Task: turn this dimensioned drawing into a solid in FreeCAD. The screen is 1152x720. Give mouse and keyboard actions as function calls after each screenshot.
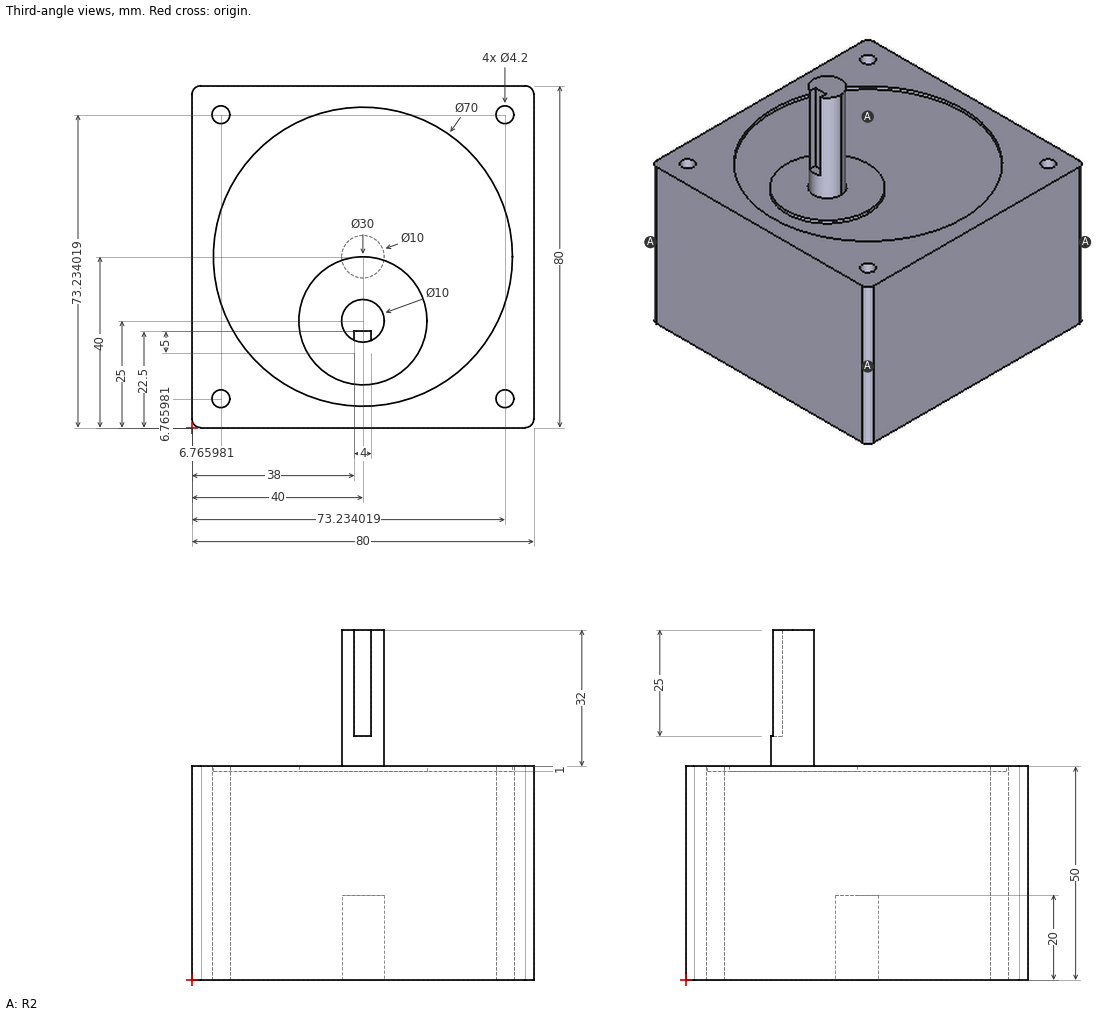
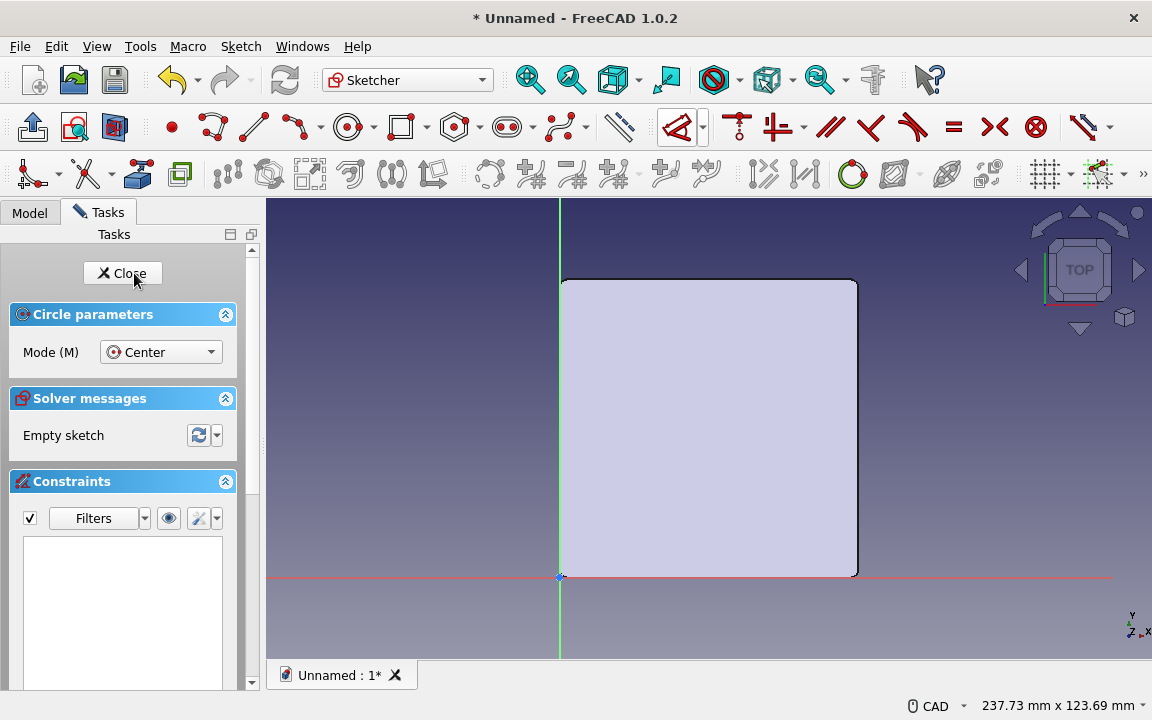
scroll(833, 305, up, 6)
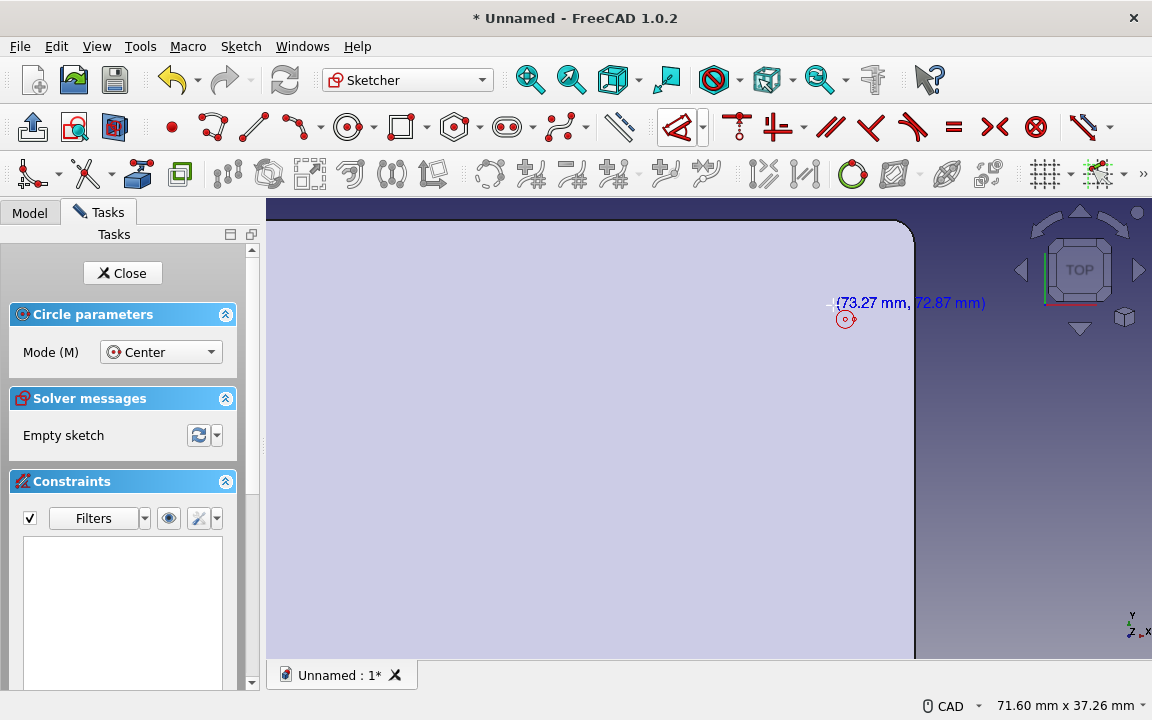
click(831, 303)
click(849, 285)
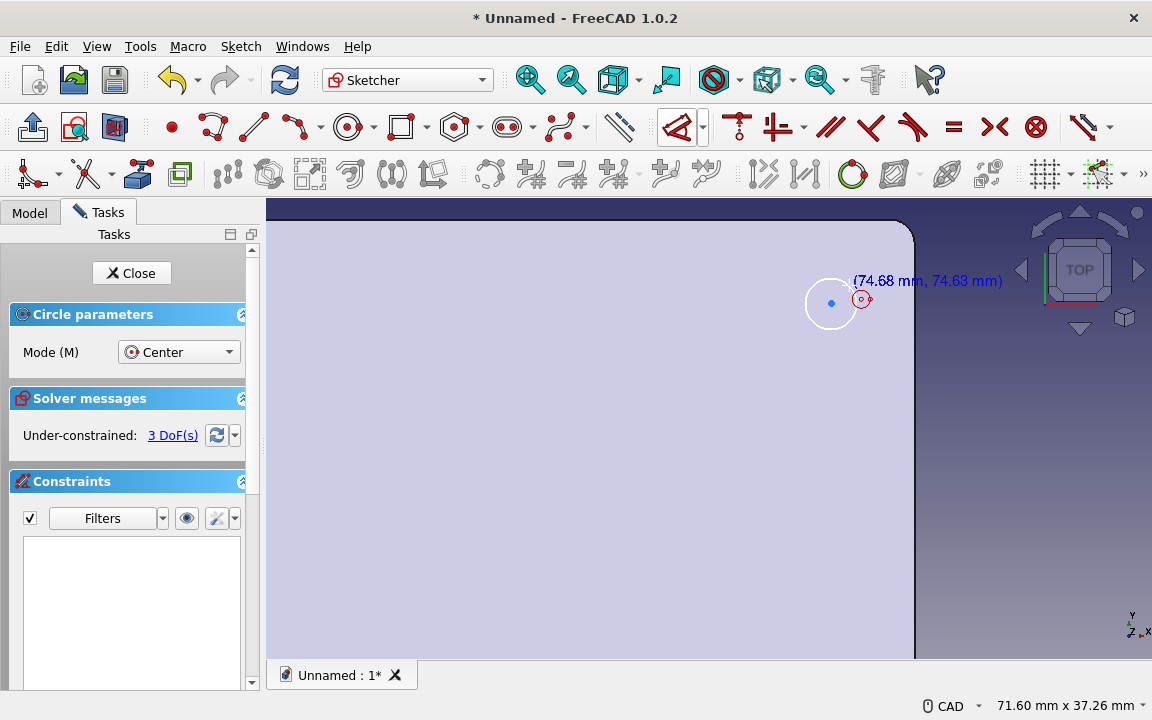
scroll(748, 293, down, 6)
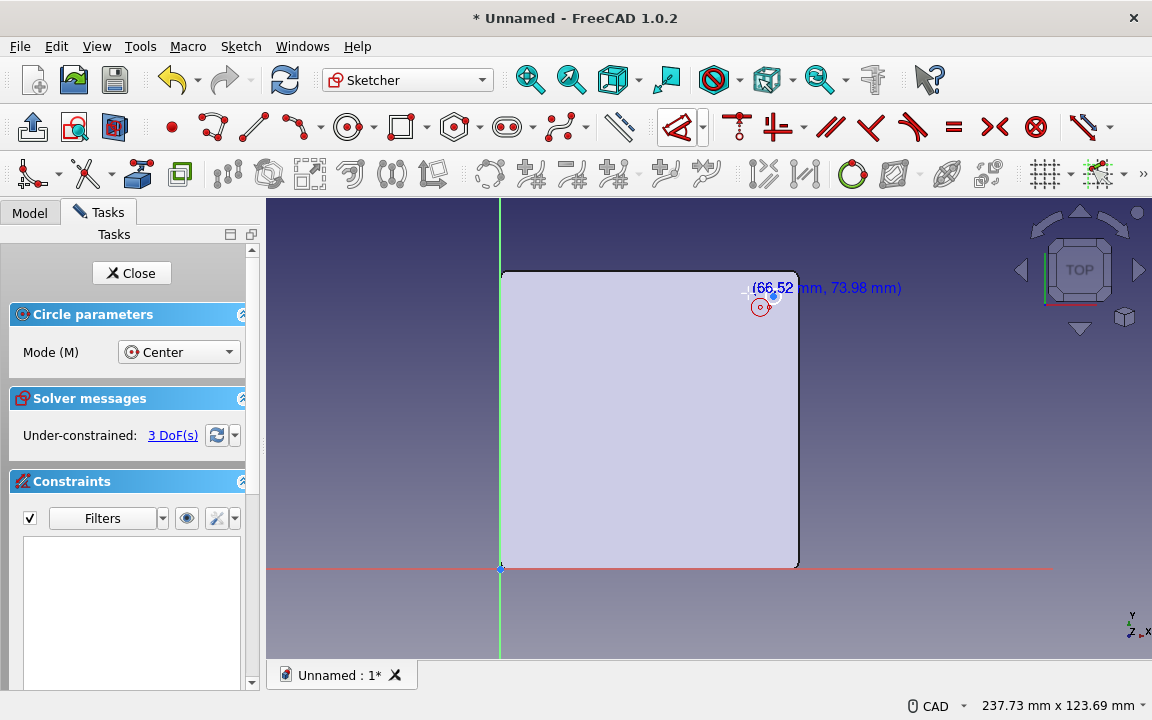
scroll(526, 296, up, 6)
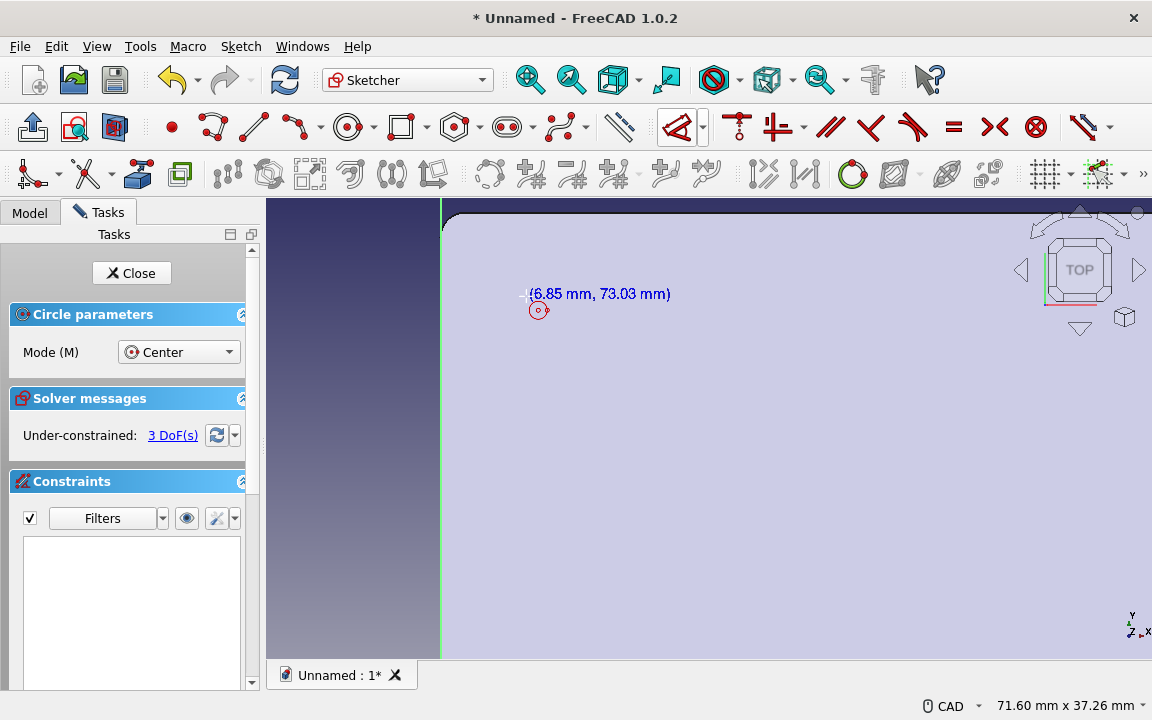
click(524, 296)
click(543, 278)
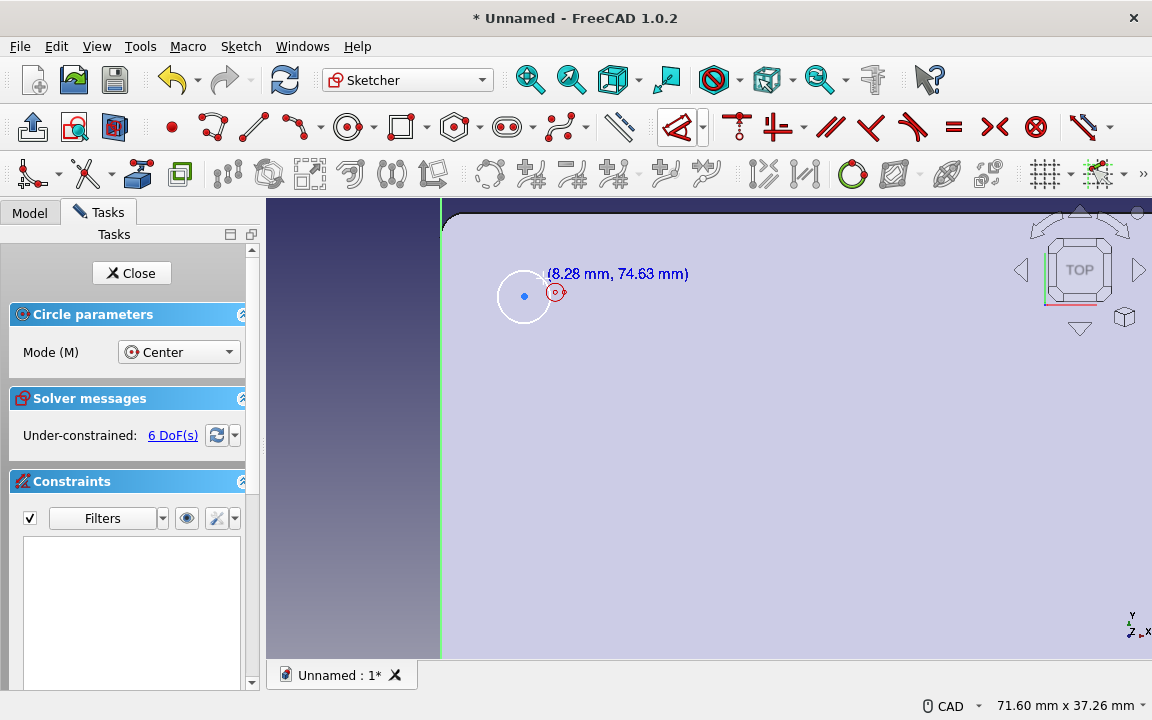
scroll(526, 296, down, 6)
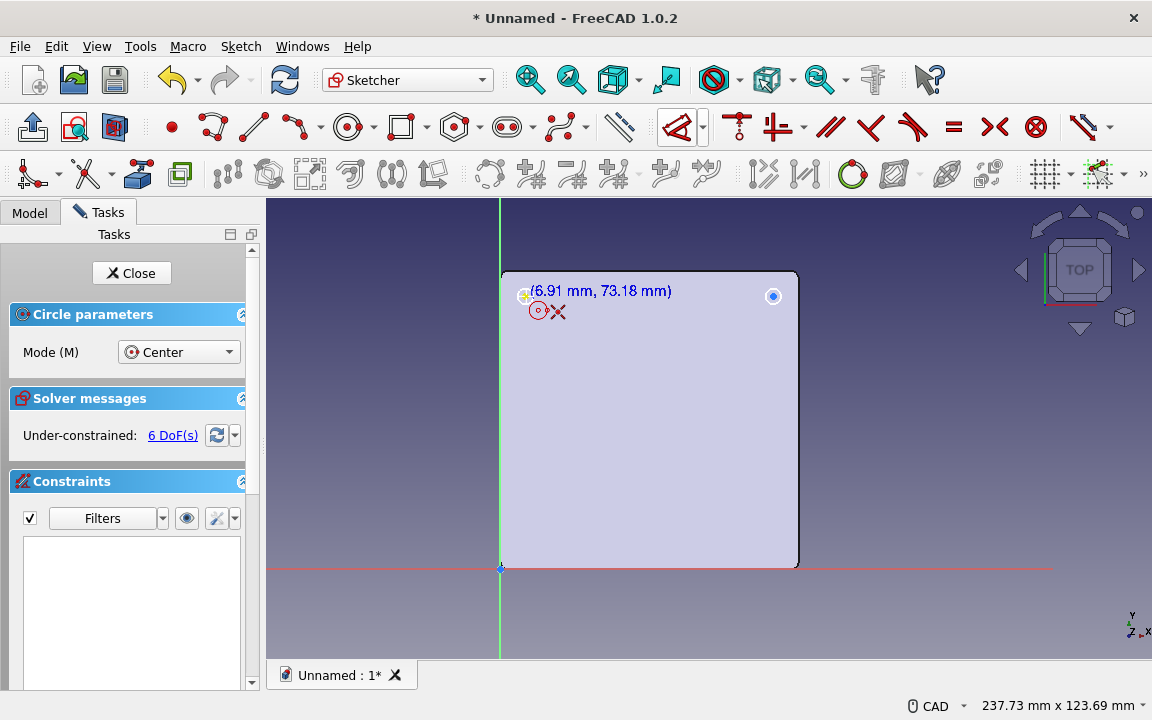
scroll(526, 544, up, 6)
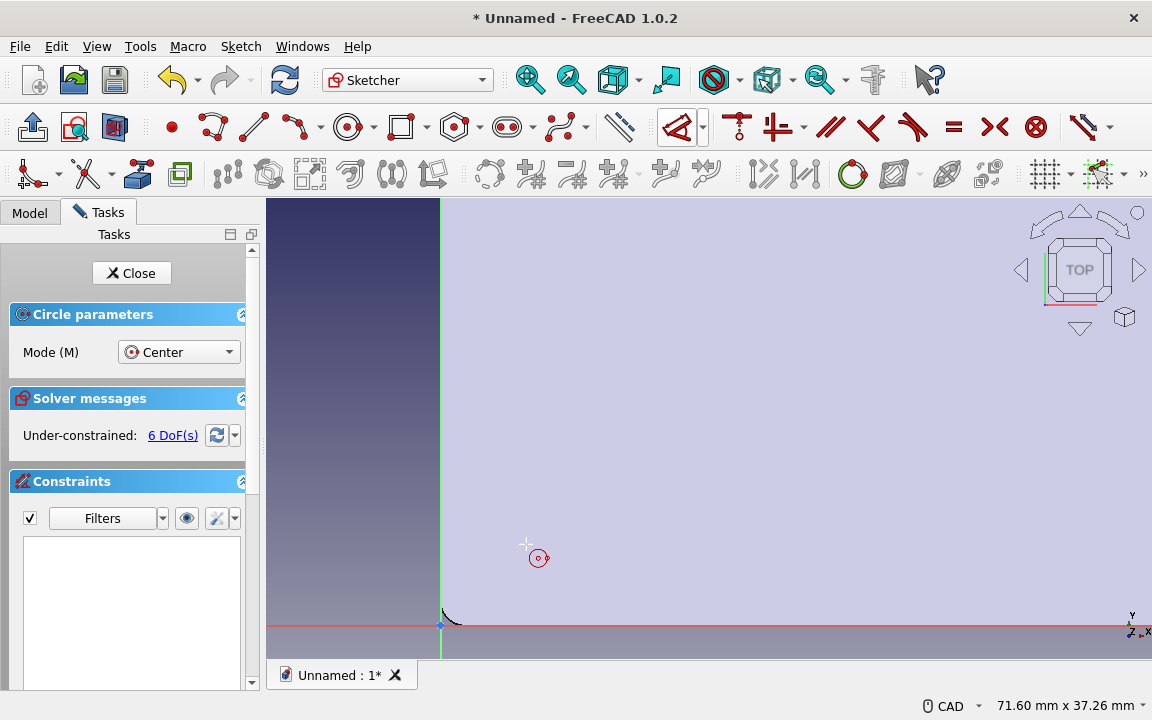
click(524, 542)
click(543, 524)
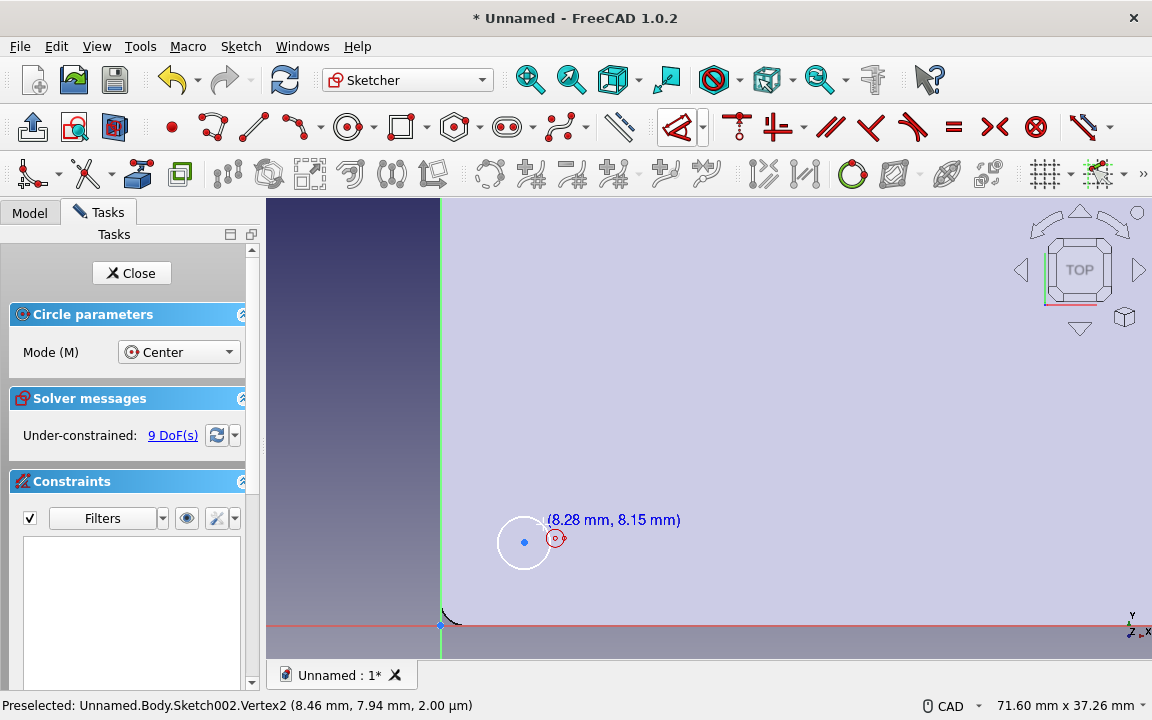
scroll(526, 544, down, 6)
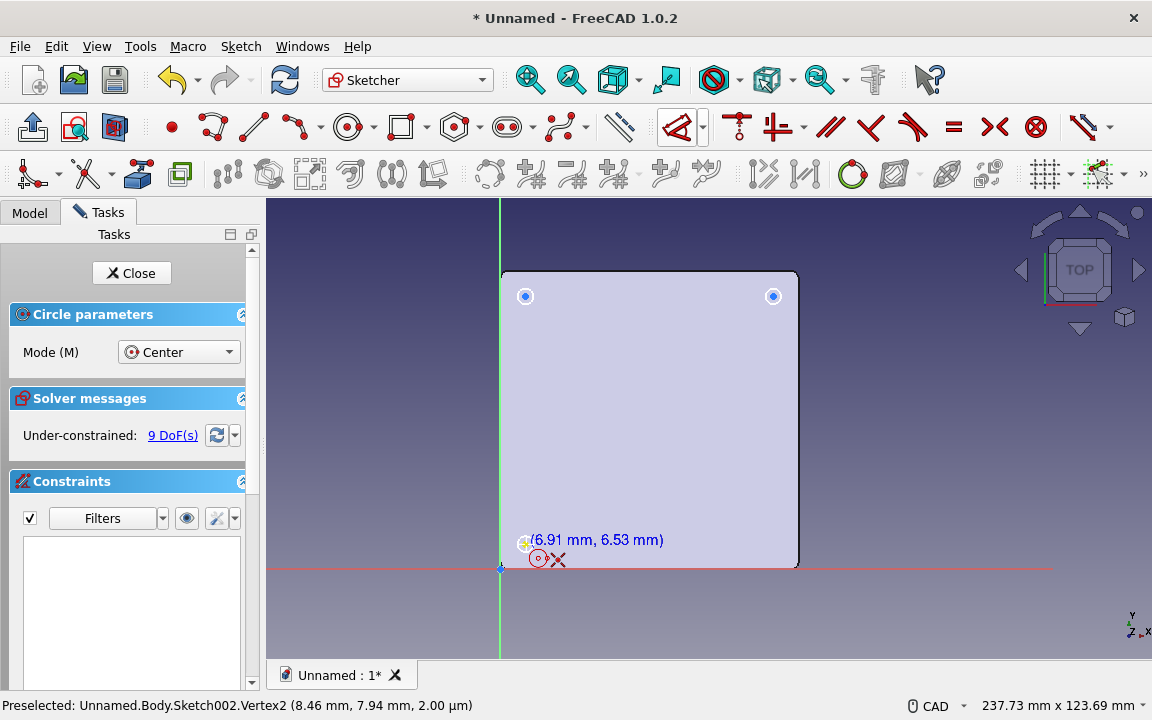
scroll(773, 544, up, 6)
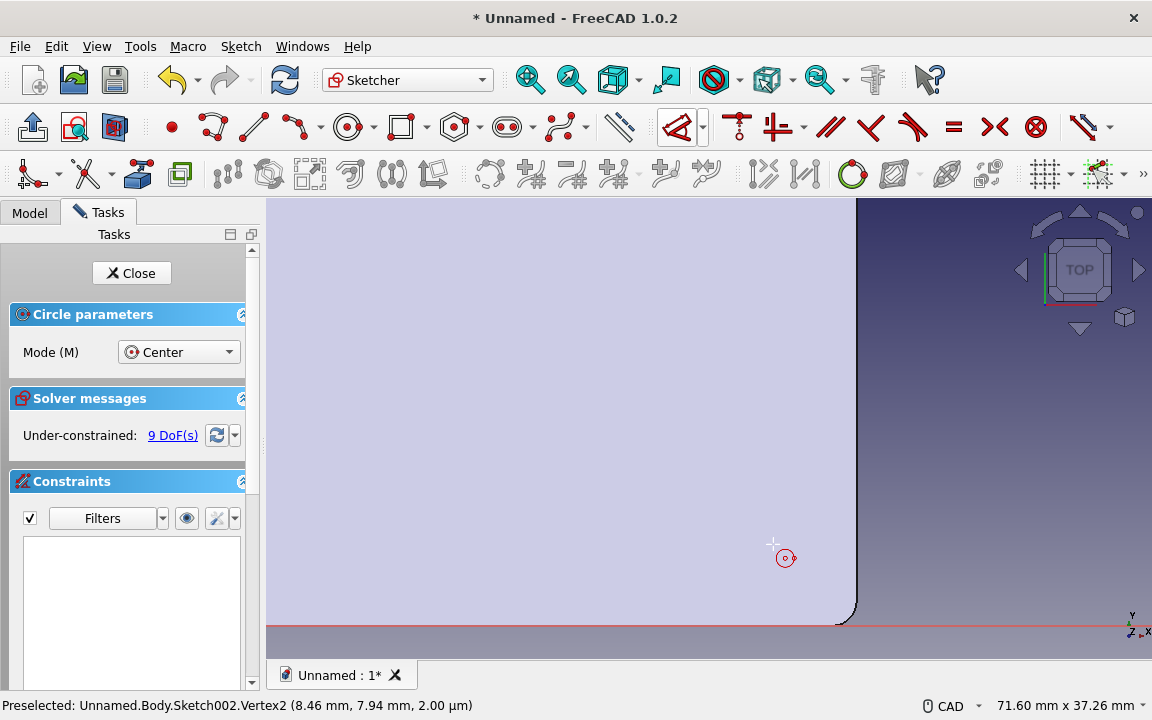
click(773, 542)
click(791, 524)
key(Escape)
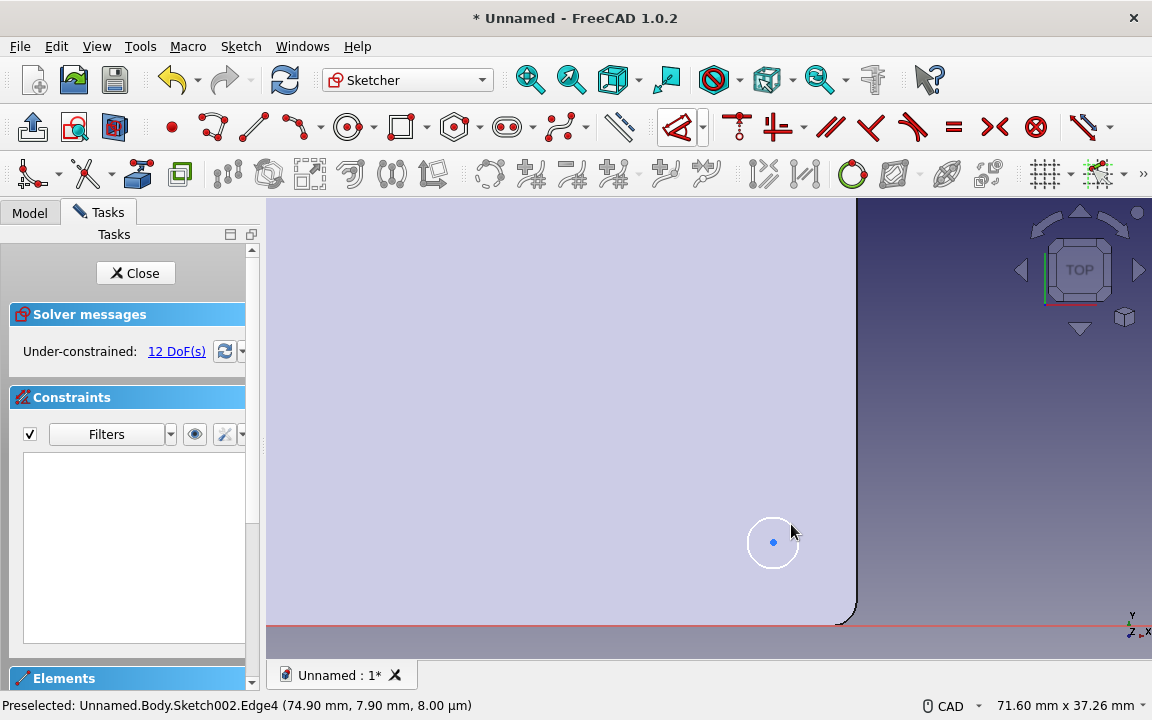
scroll(773, 544, down, 6)